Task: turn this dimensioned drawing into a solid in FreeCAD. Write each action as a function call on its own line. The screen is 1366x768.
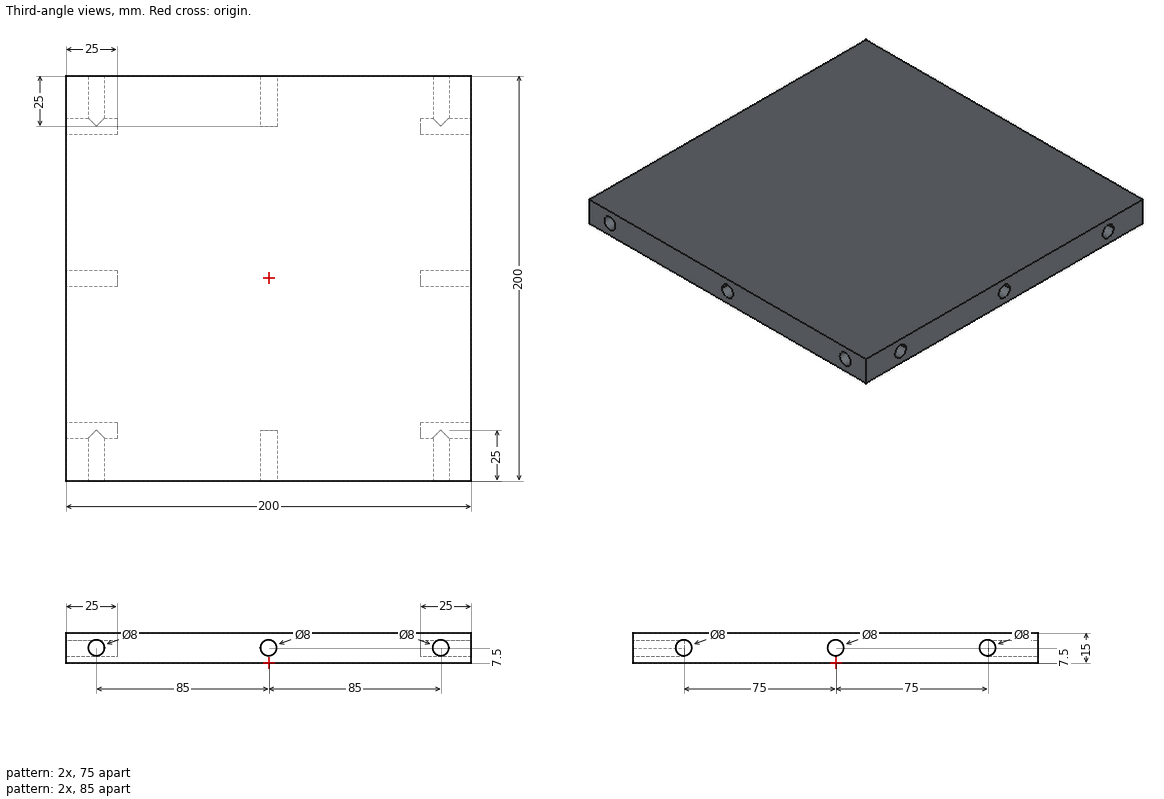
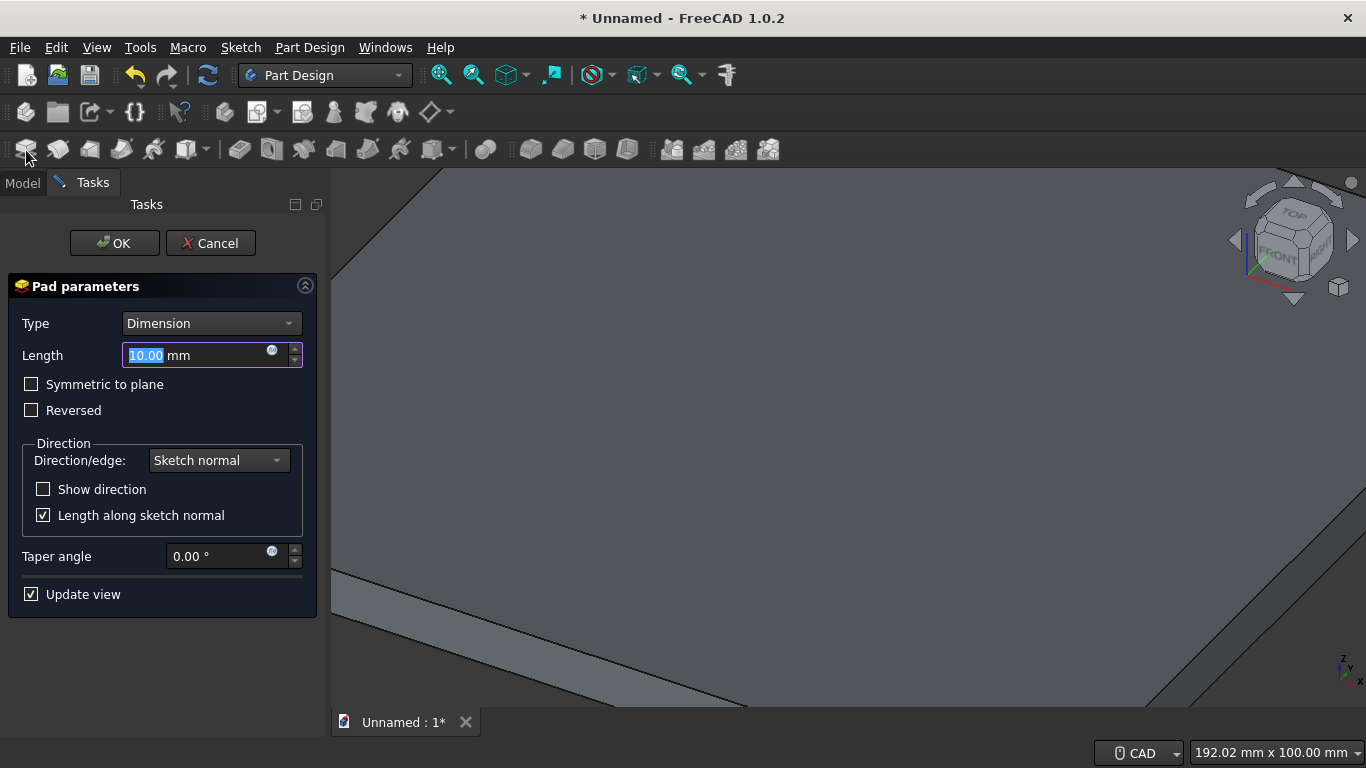
text(15)
key(Tab)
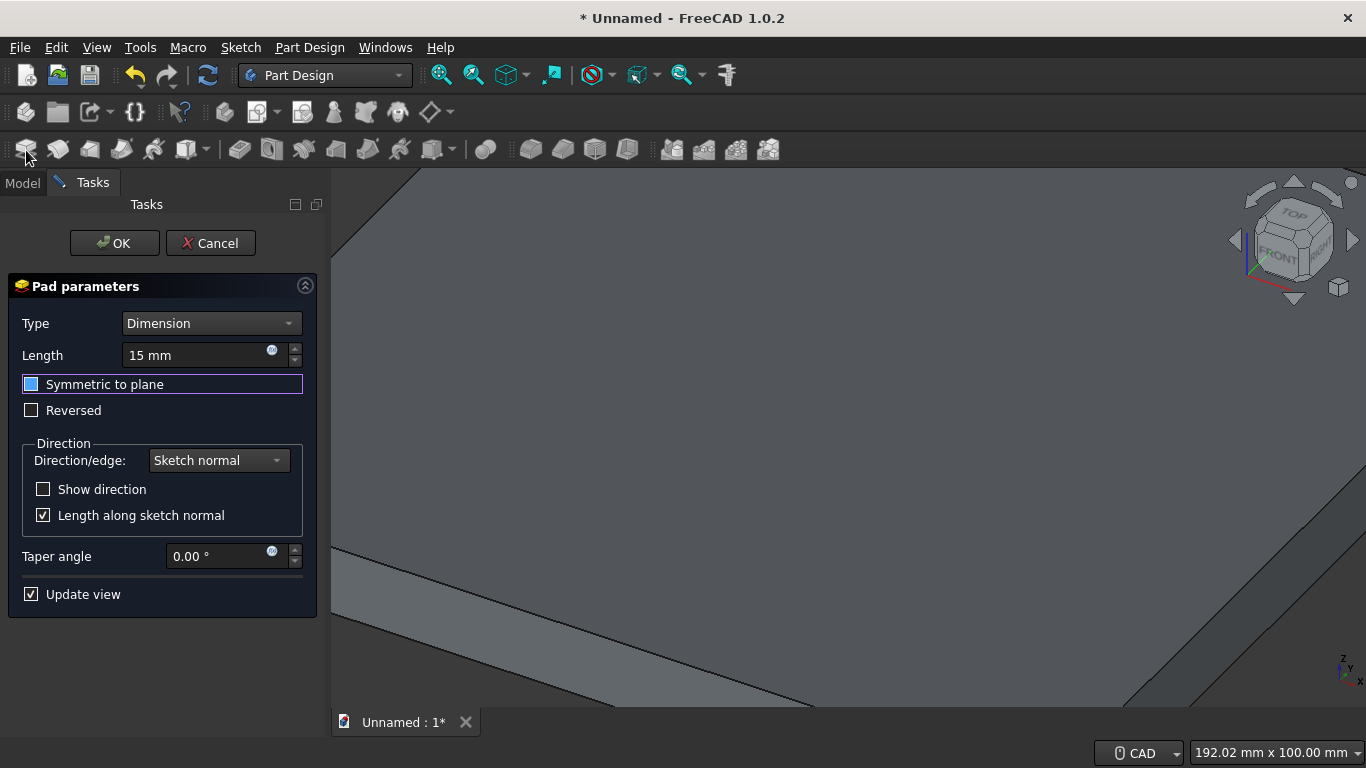
click(115, 243)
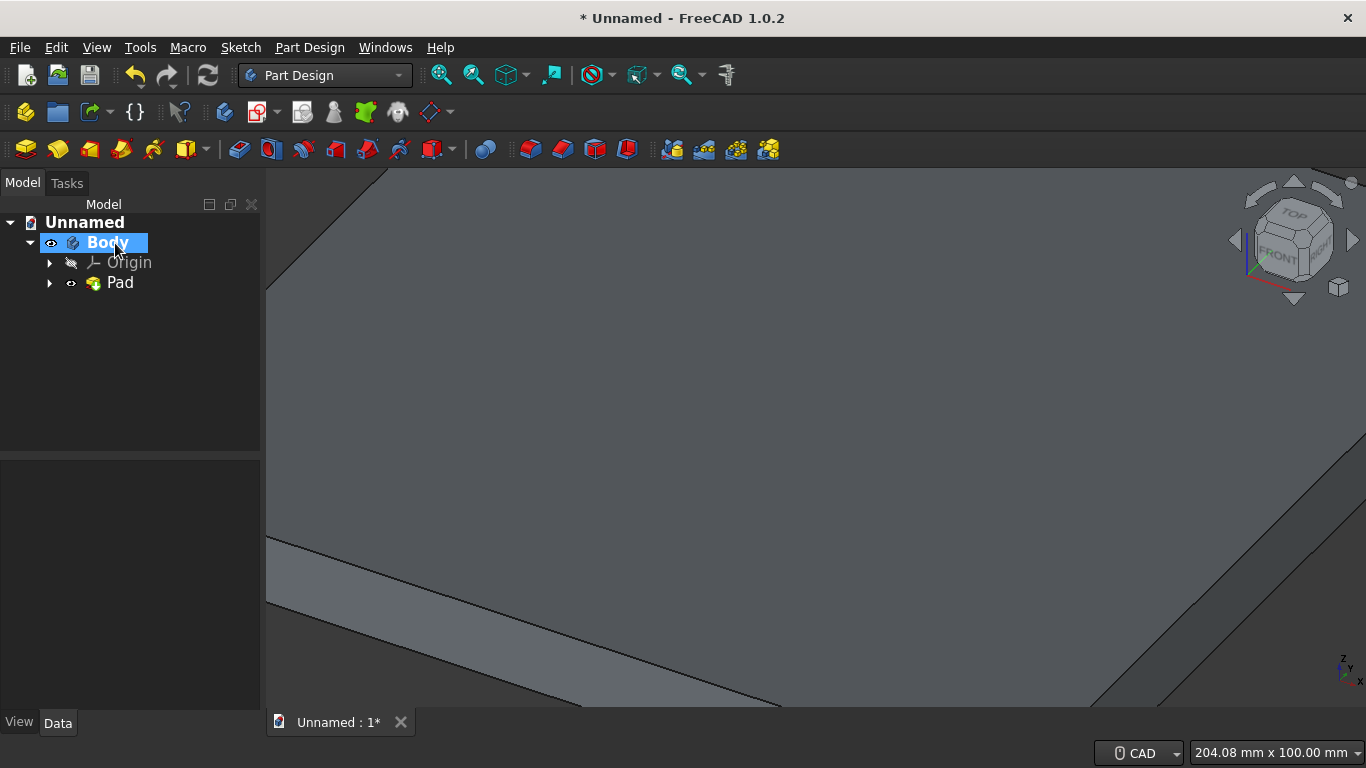
key(v)
key(f)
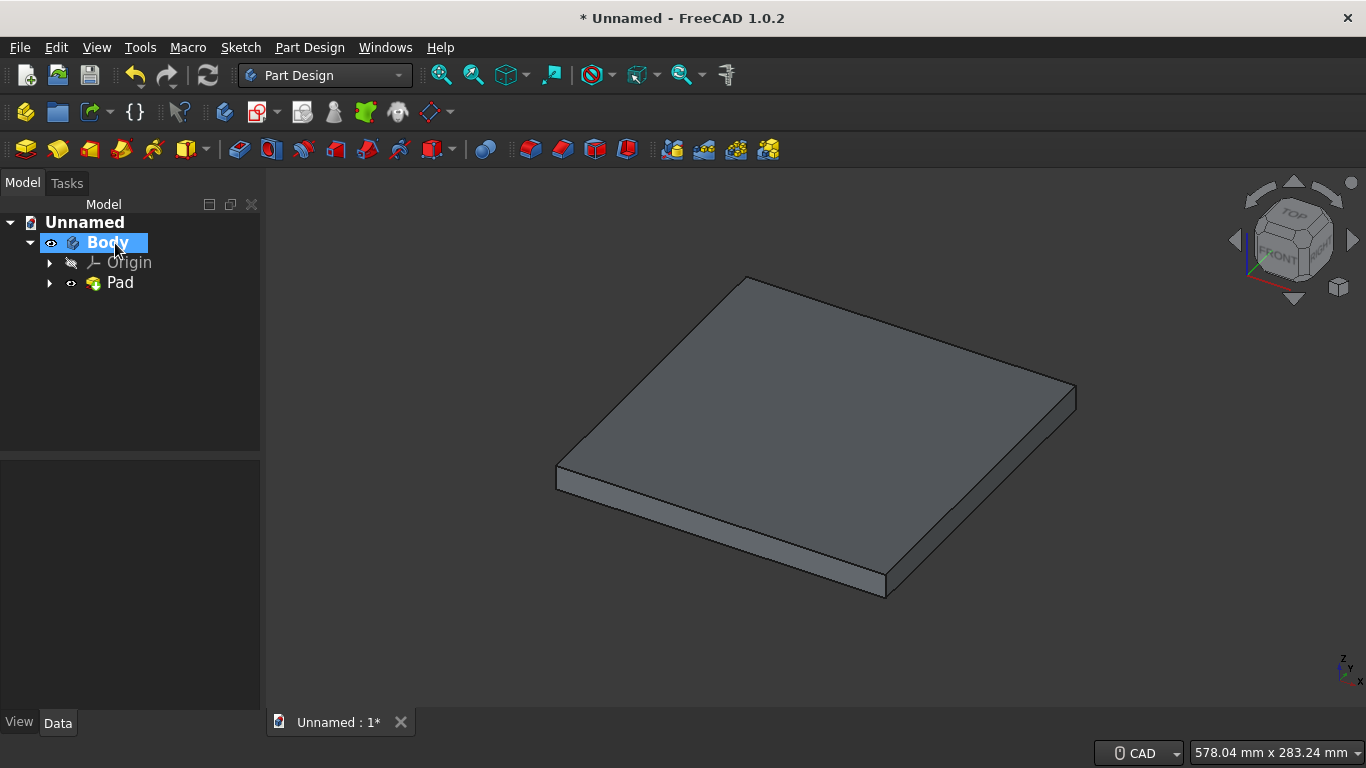
key(0)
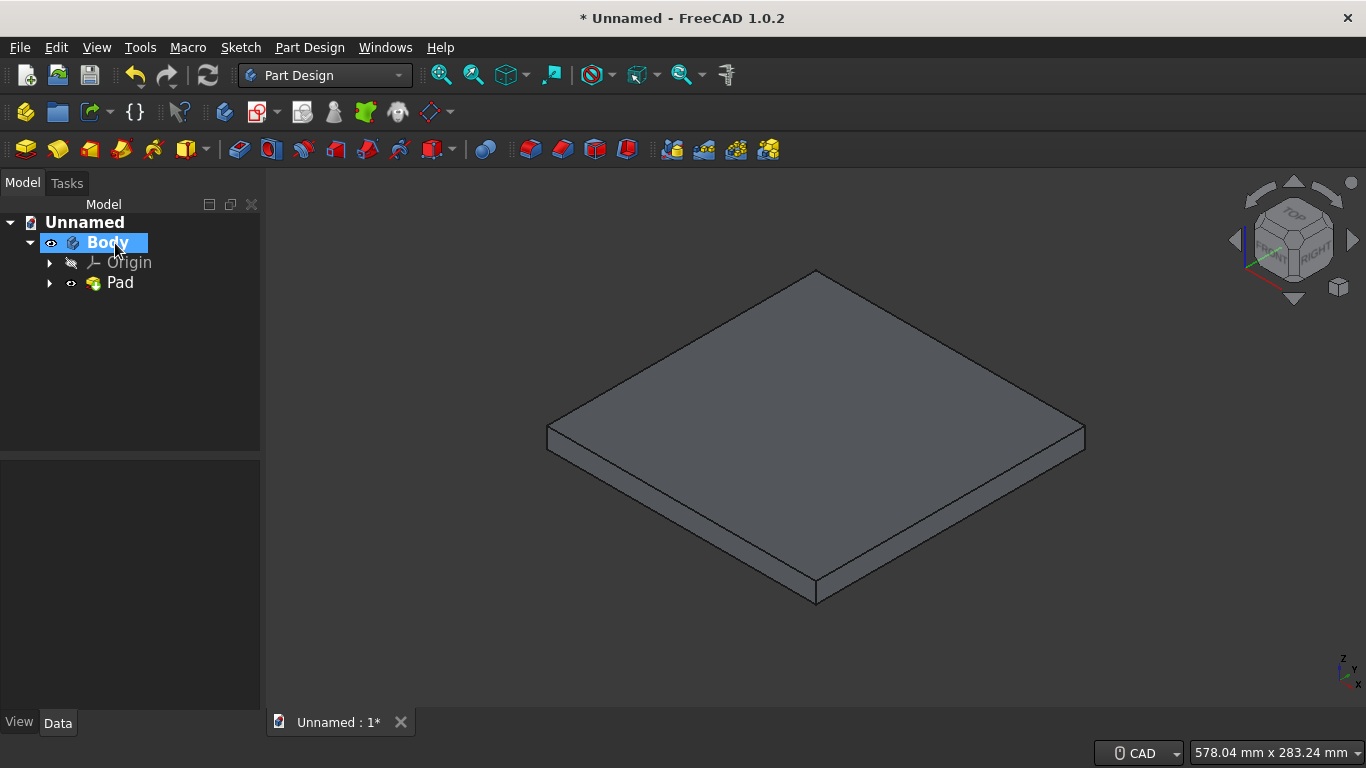
click(1066, 448)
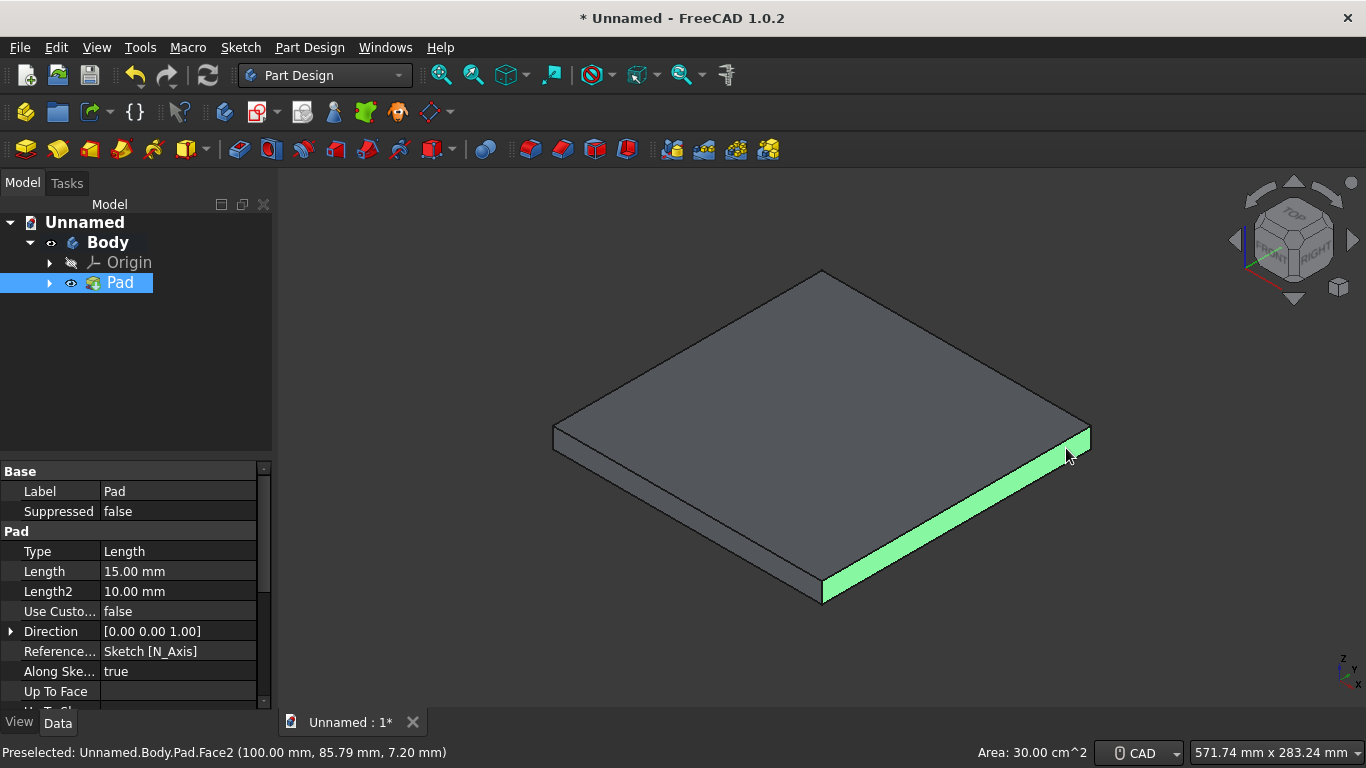
click(258, 112)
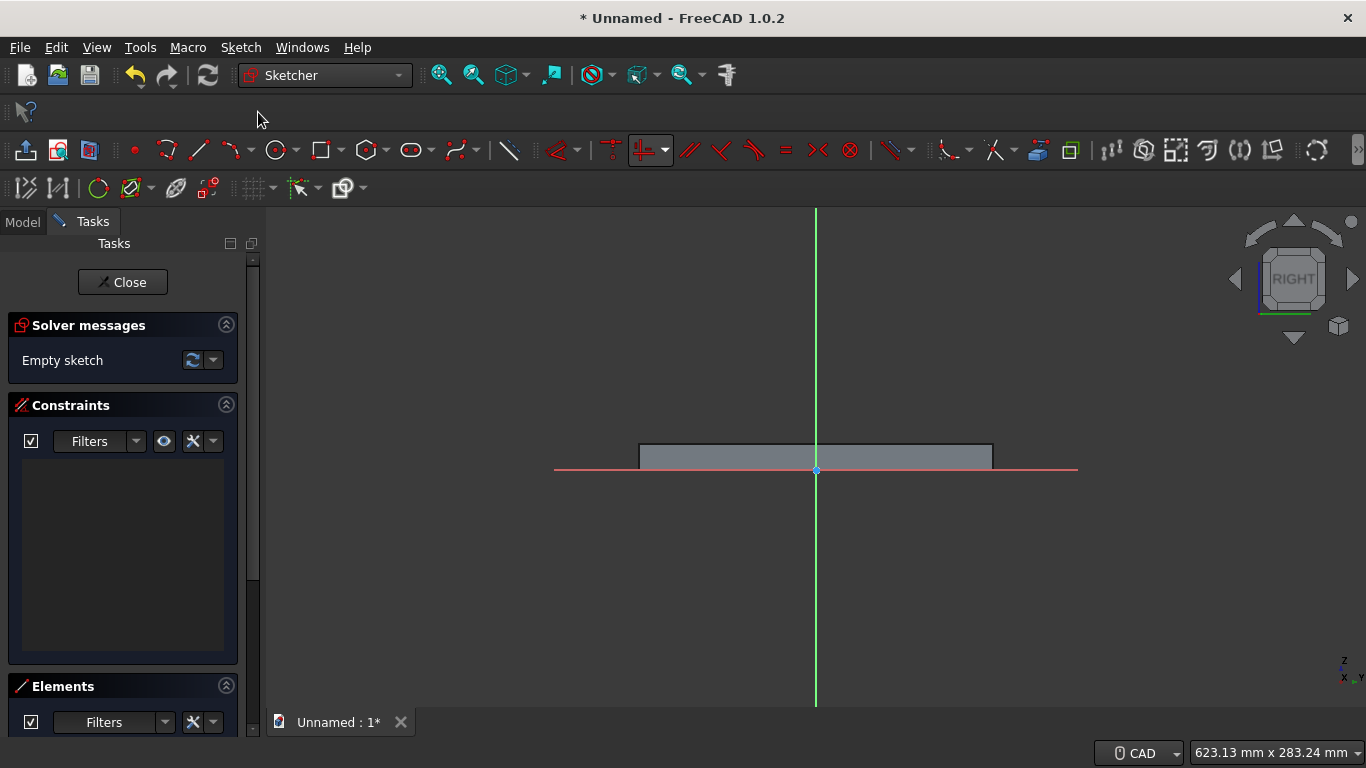
scroll(820, 460, up, 14)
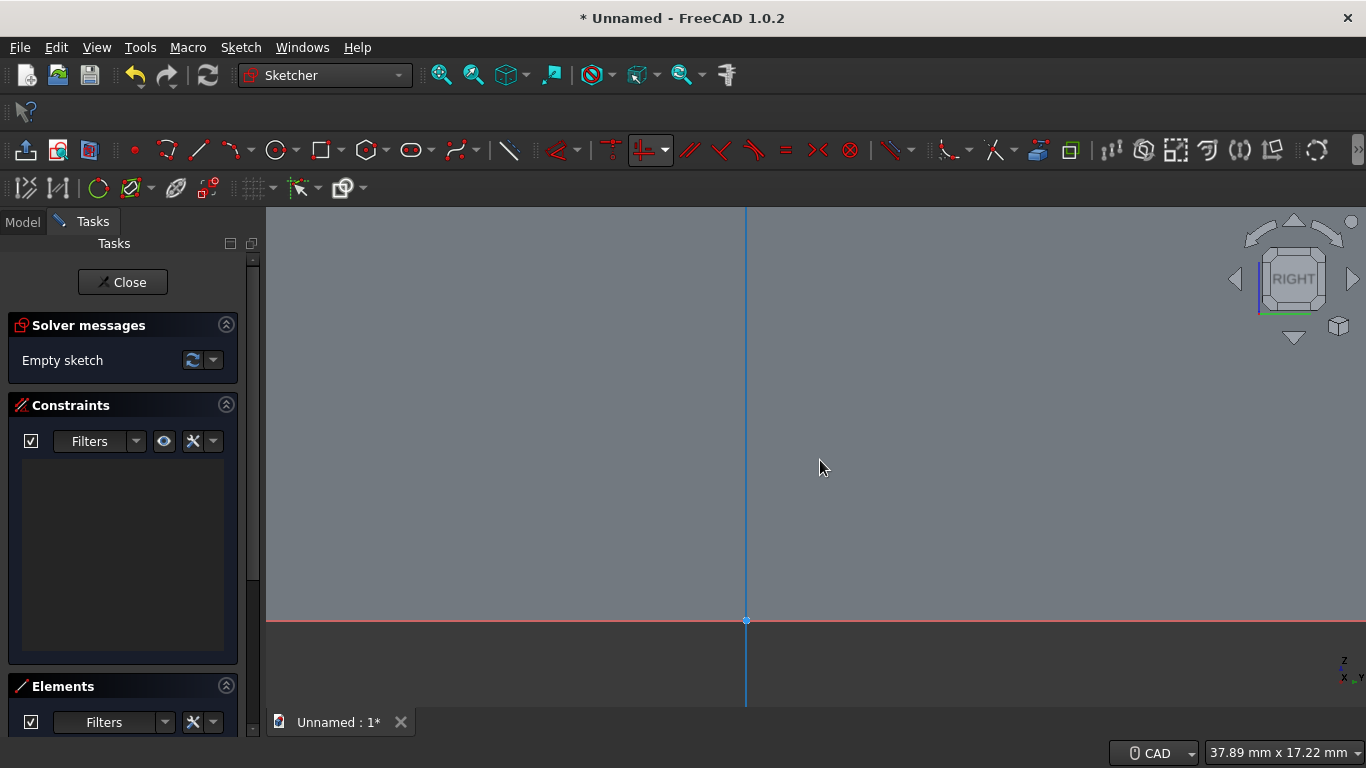
key(g)
key(c)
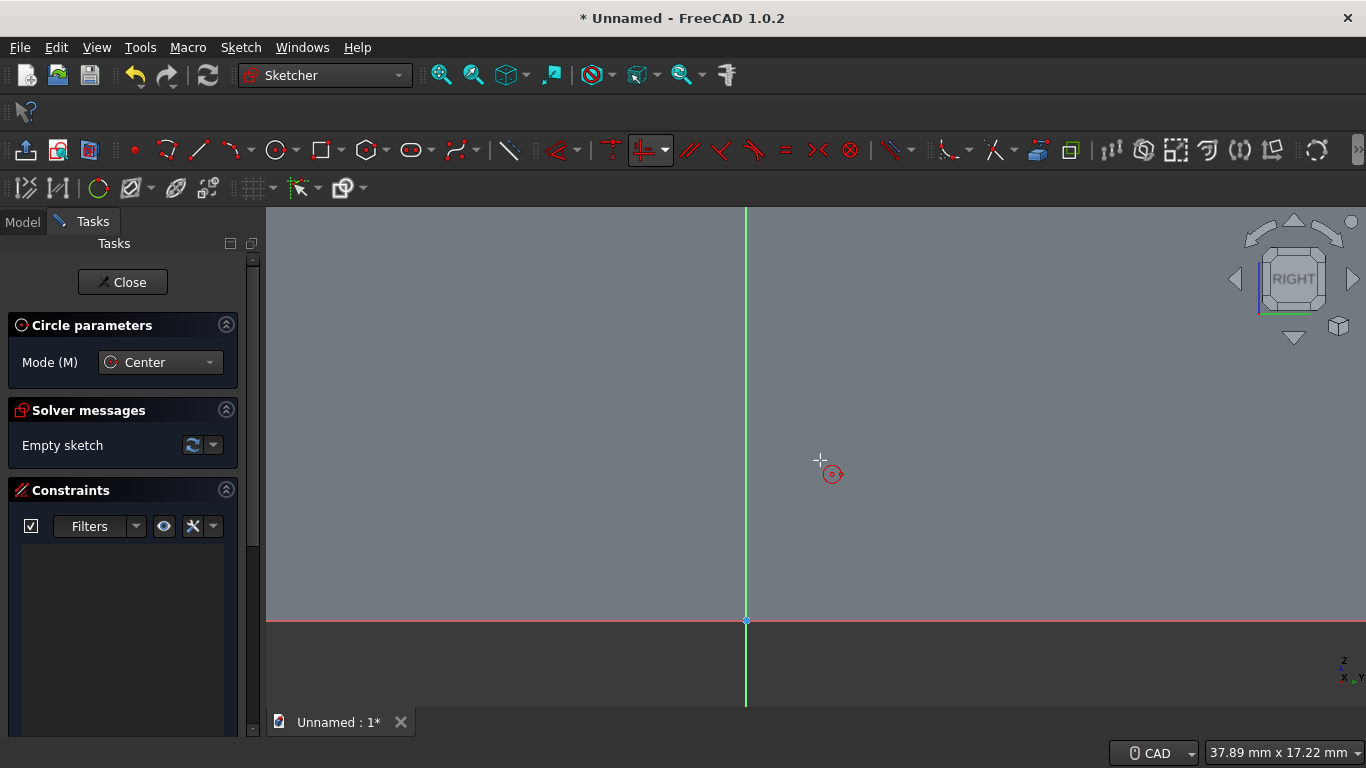
click(746, 403)
move(829, 321)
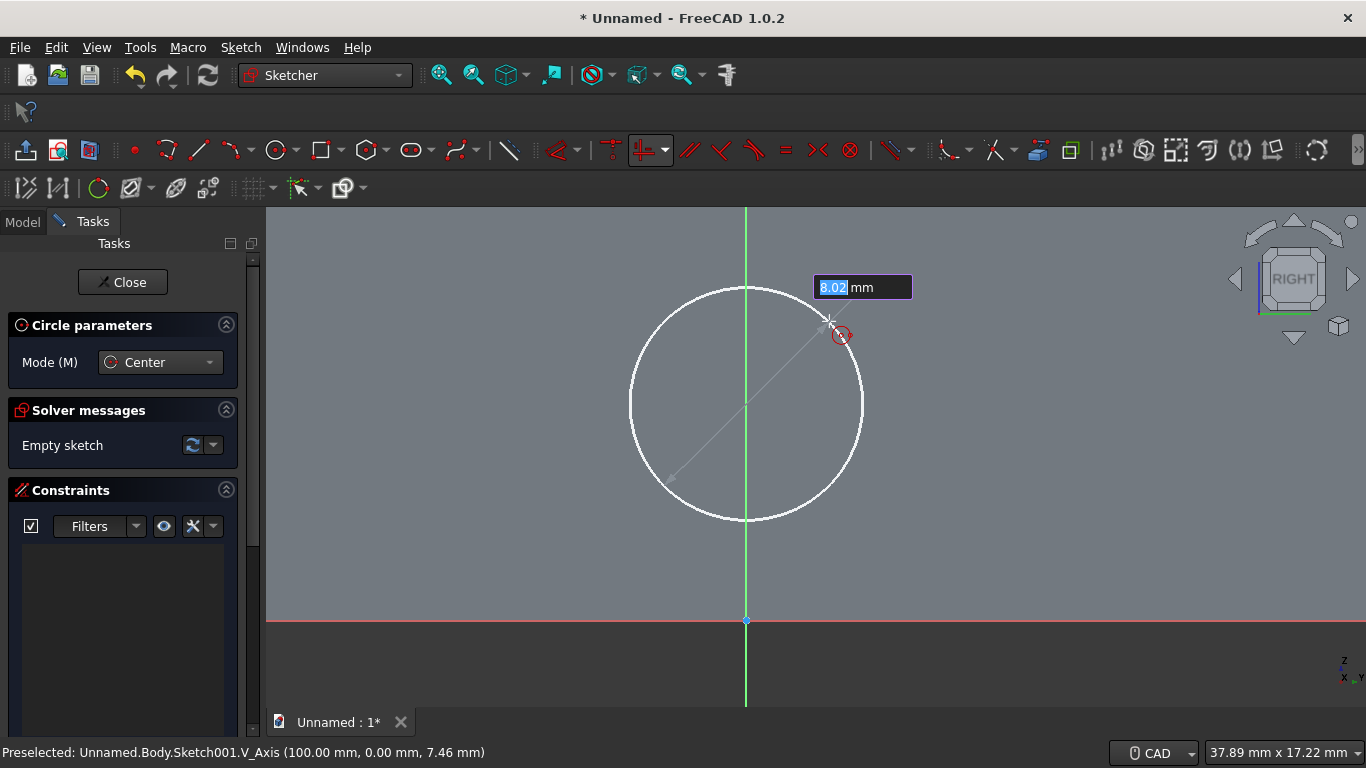
text(8)
key(Return)
key(Escape)